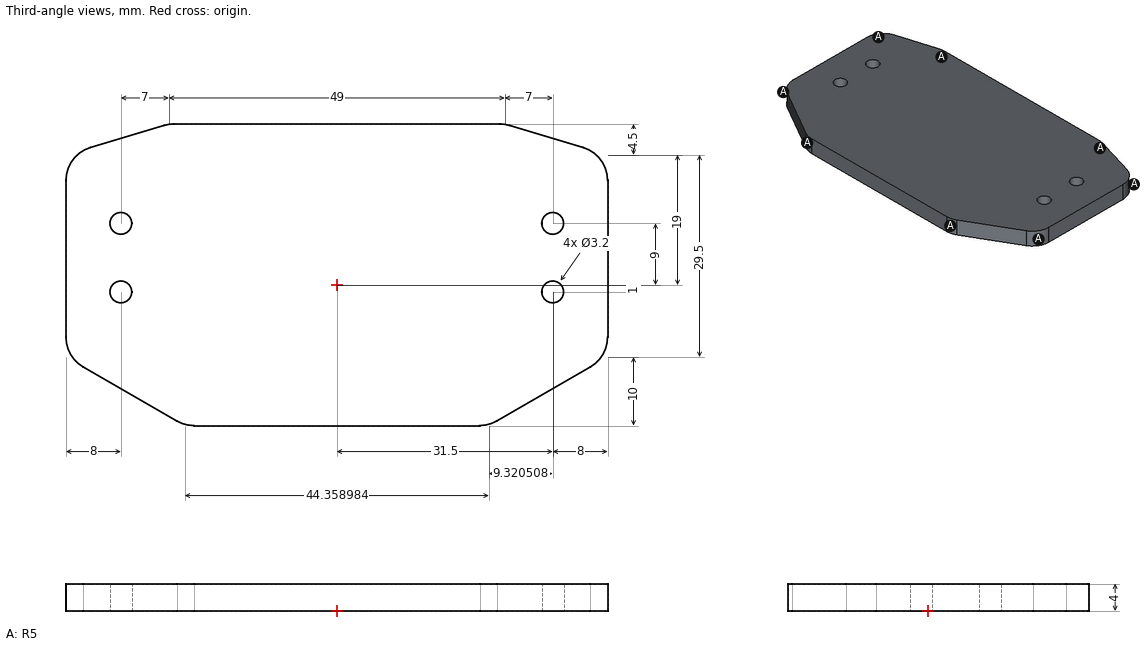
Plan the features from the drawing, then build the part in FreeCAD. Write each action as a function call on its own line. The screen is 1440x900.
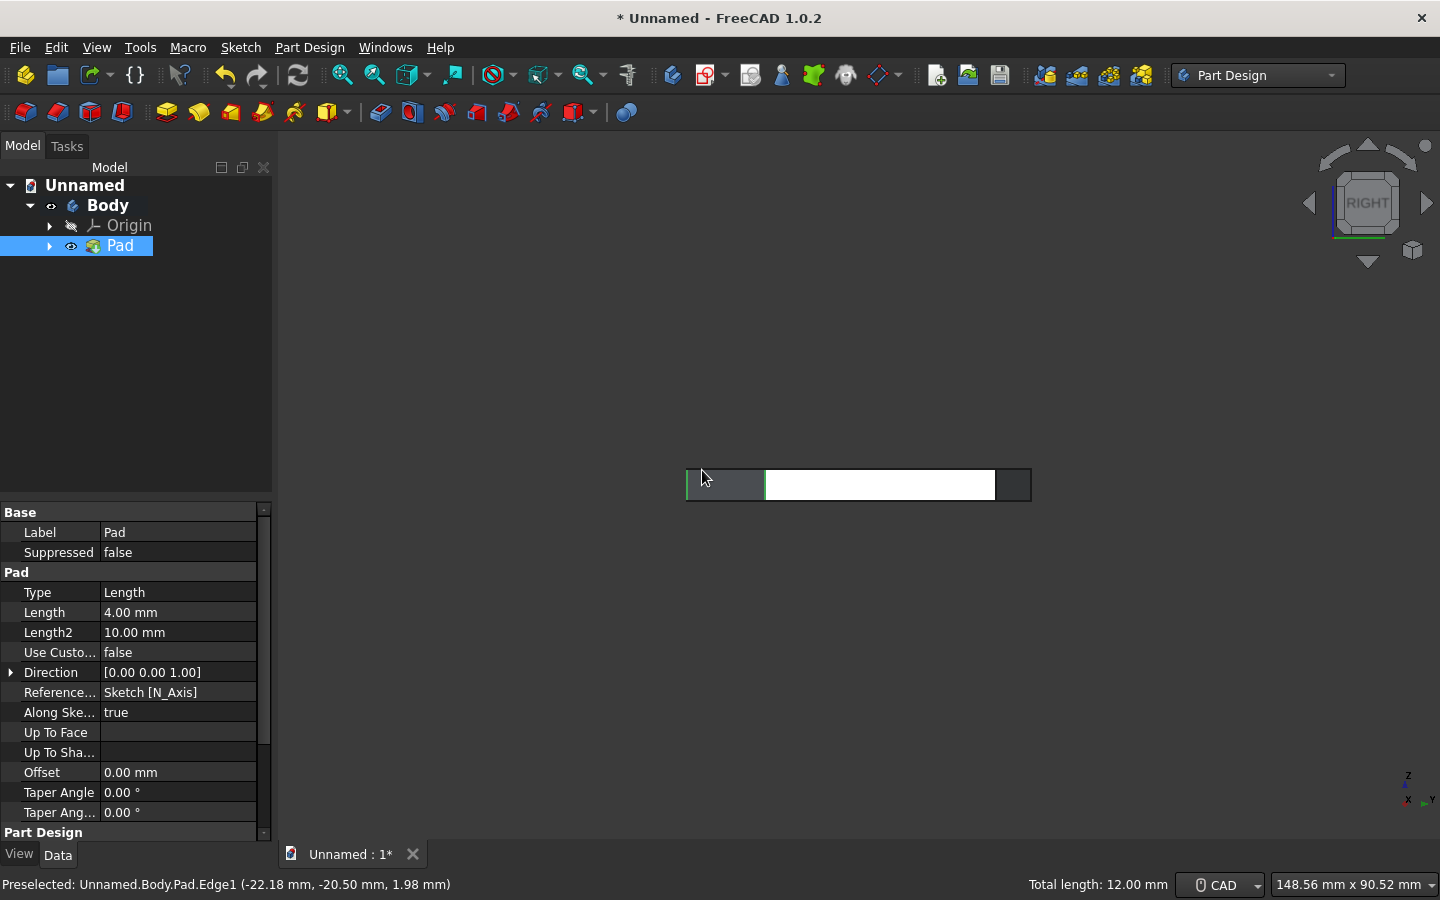
click(996, 484, ctrl)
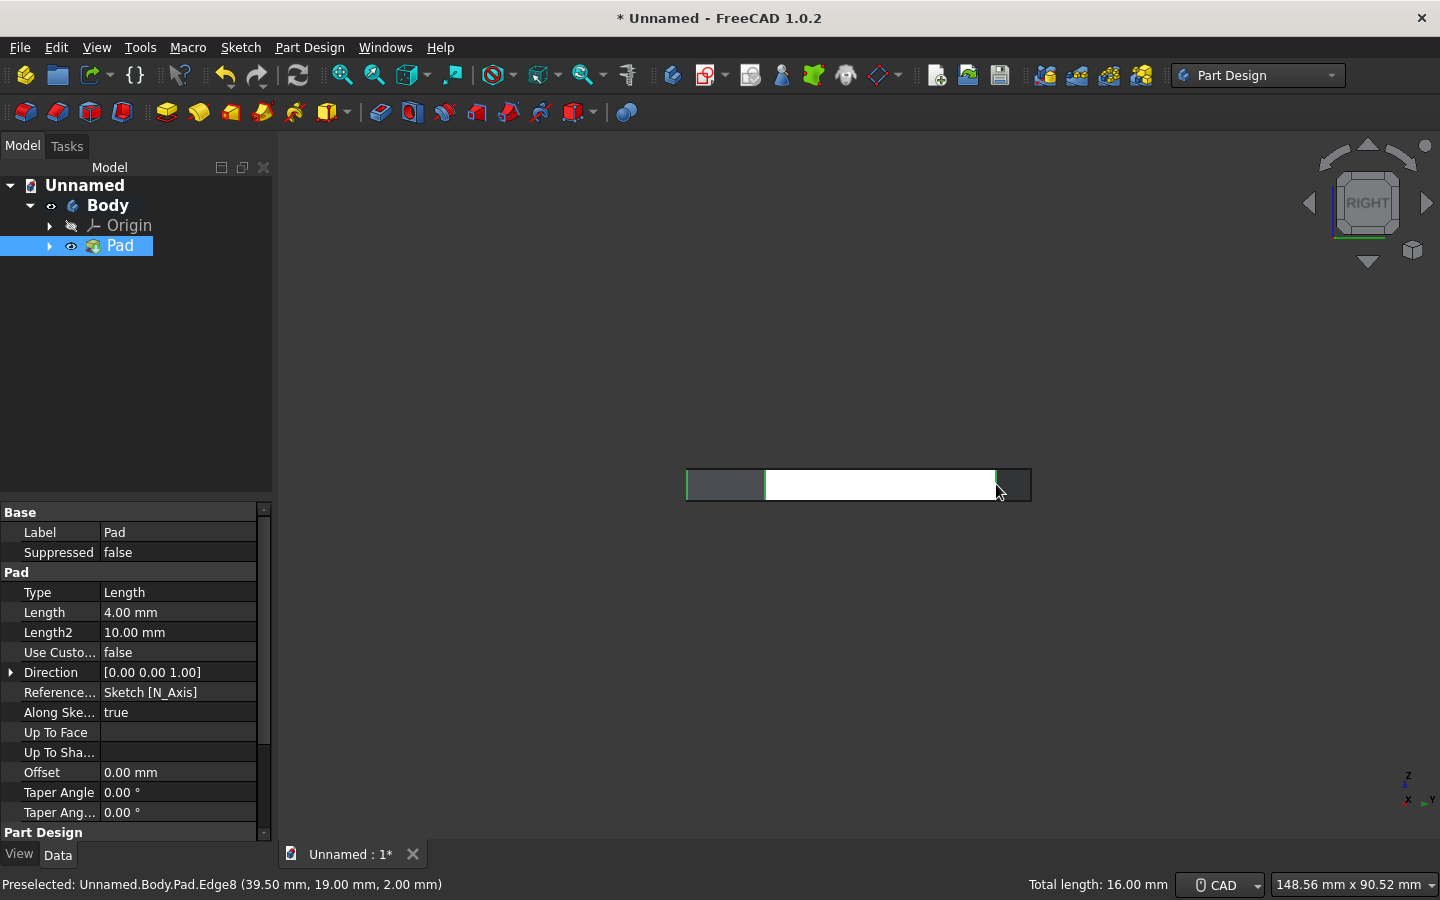
key(5)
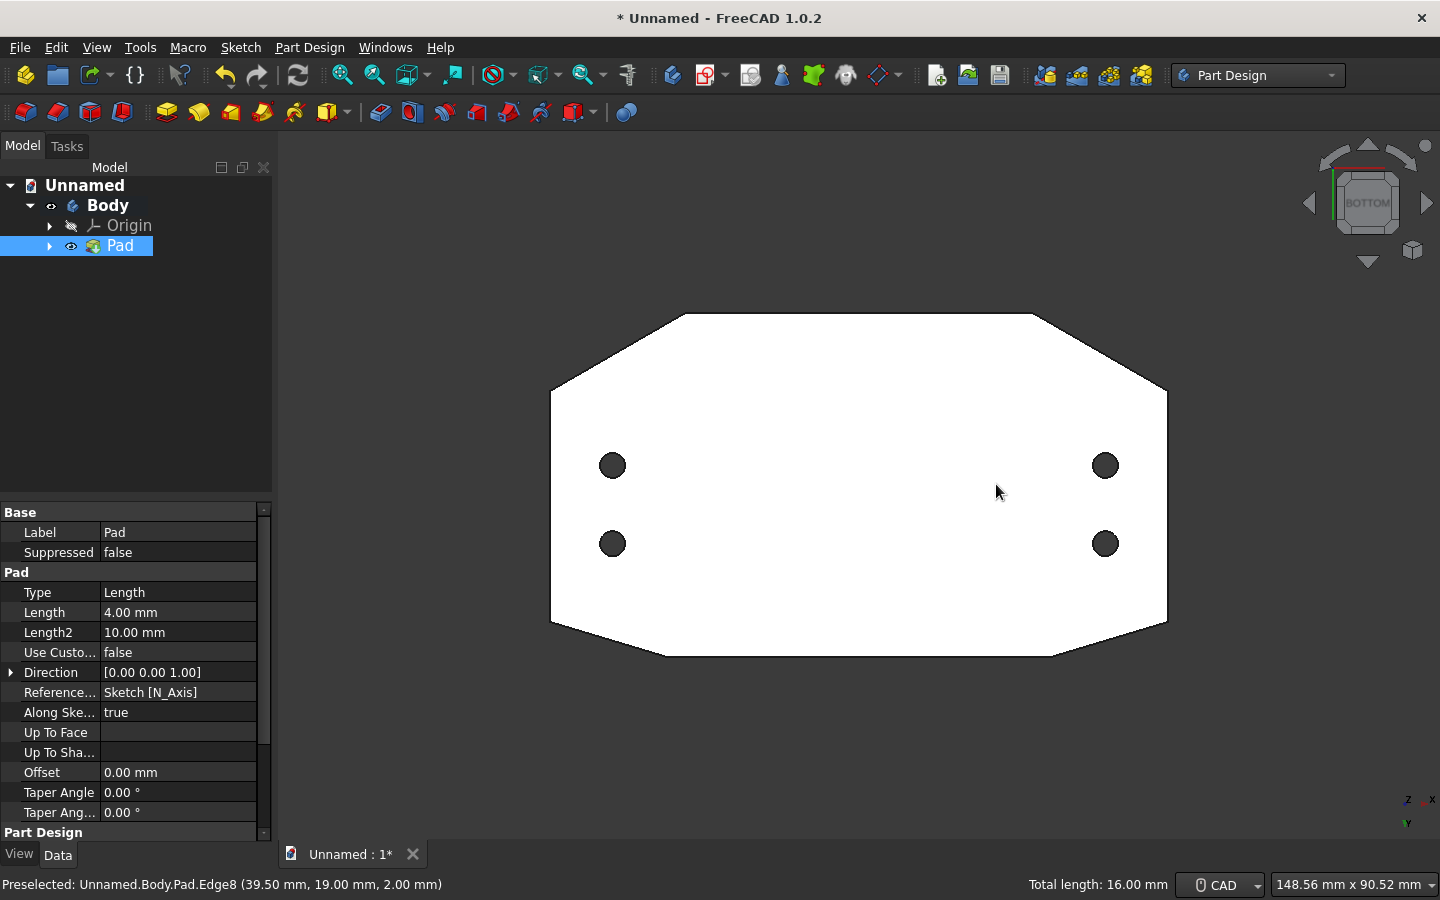
key(4)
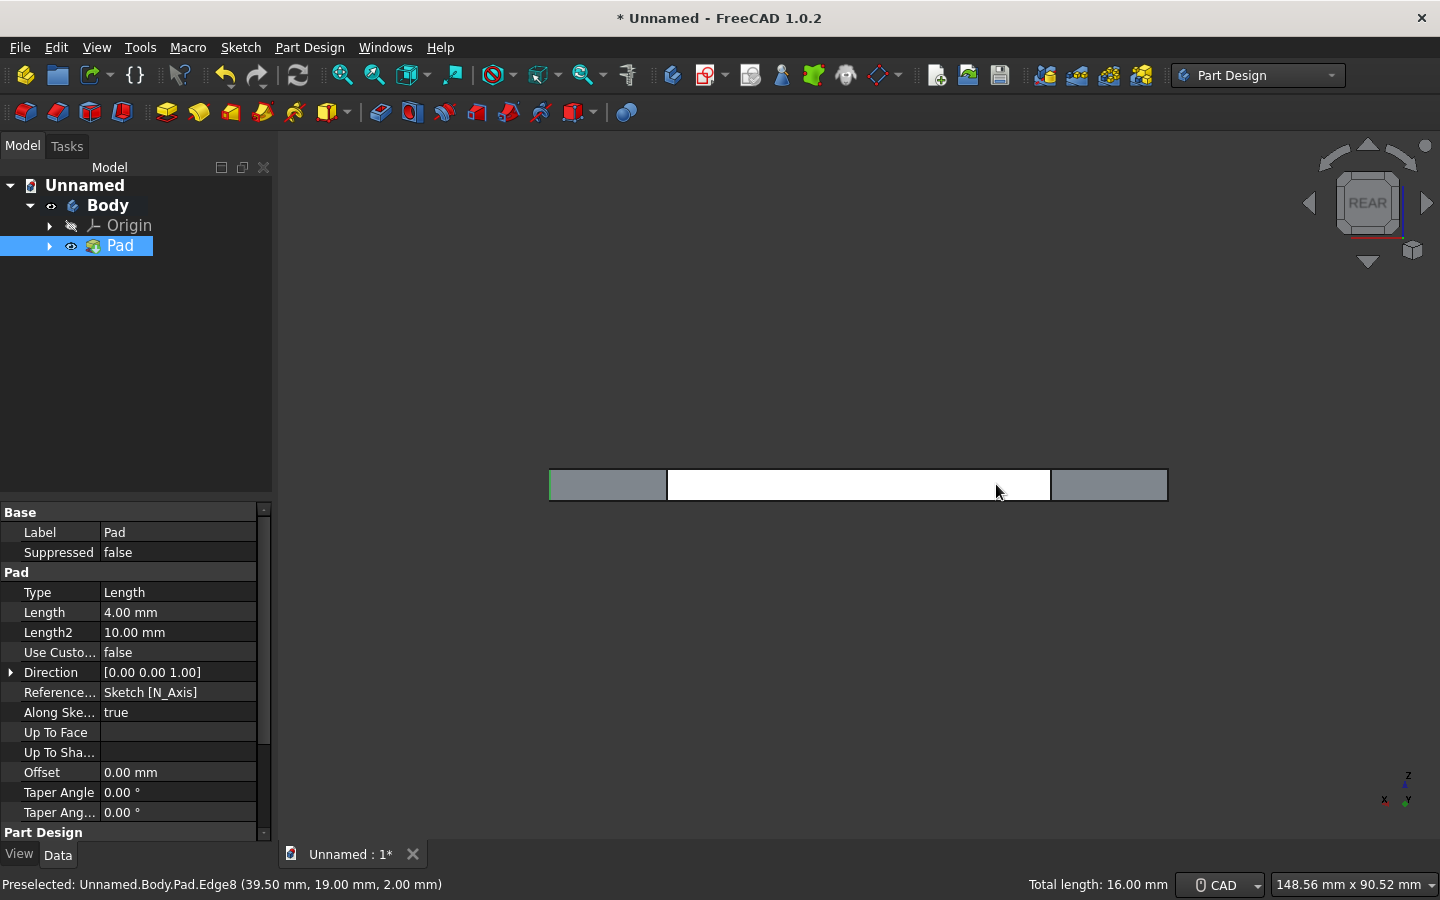
click(1051, 484, ctrl)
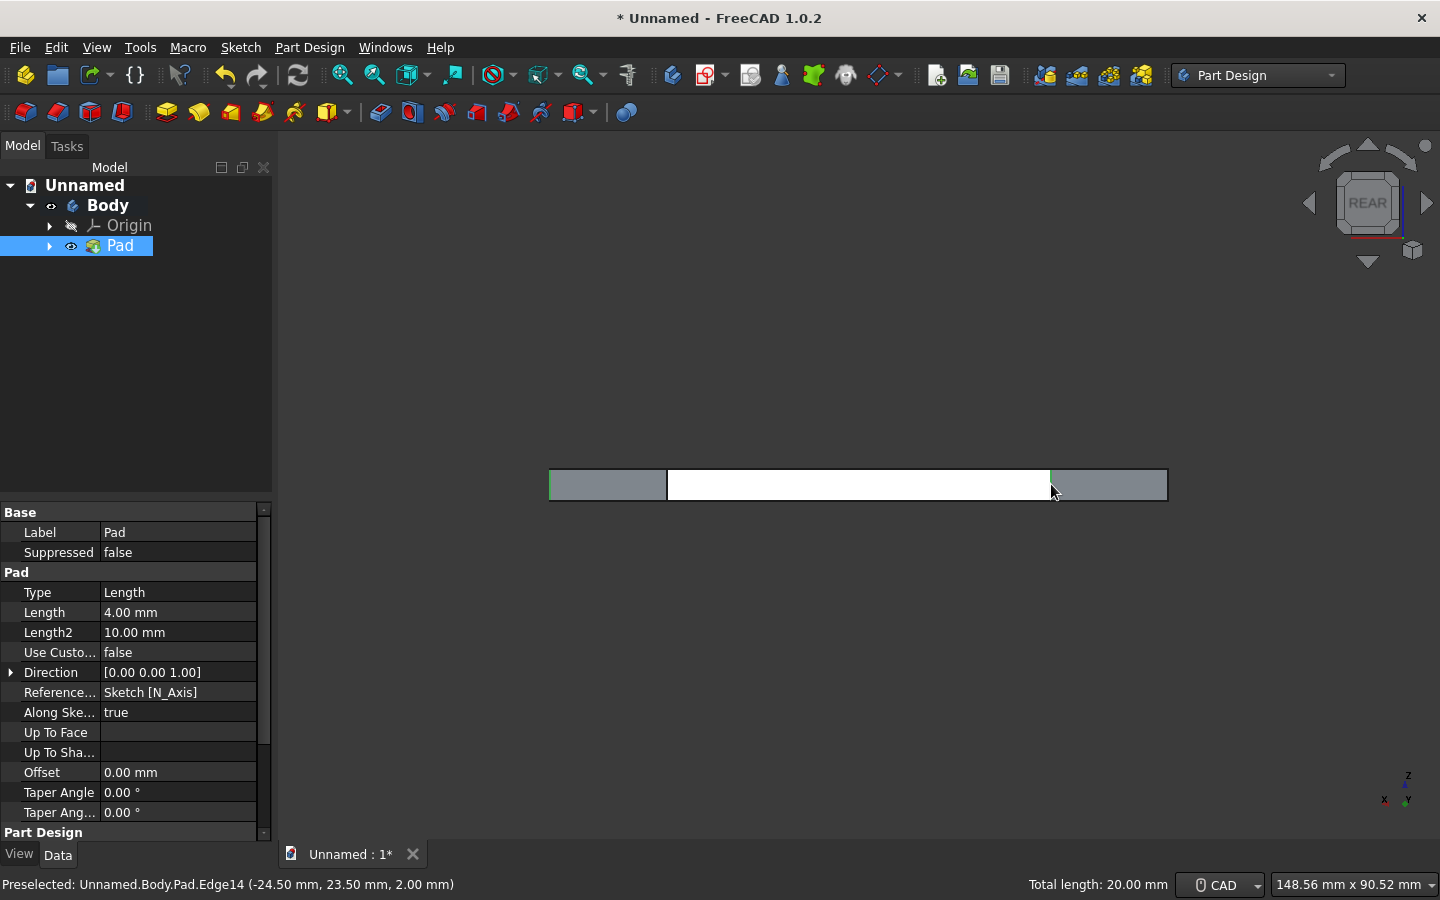
click(667, 484, ctrl)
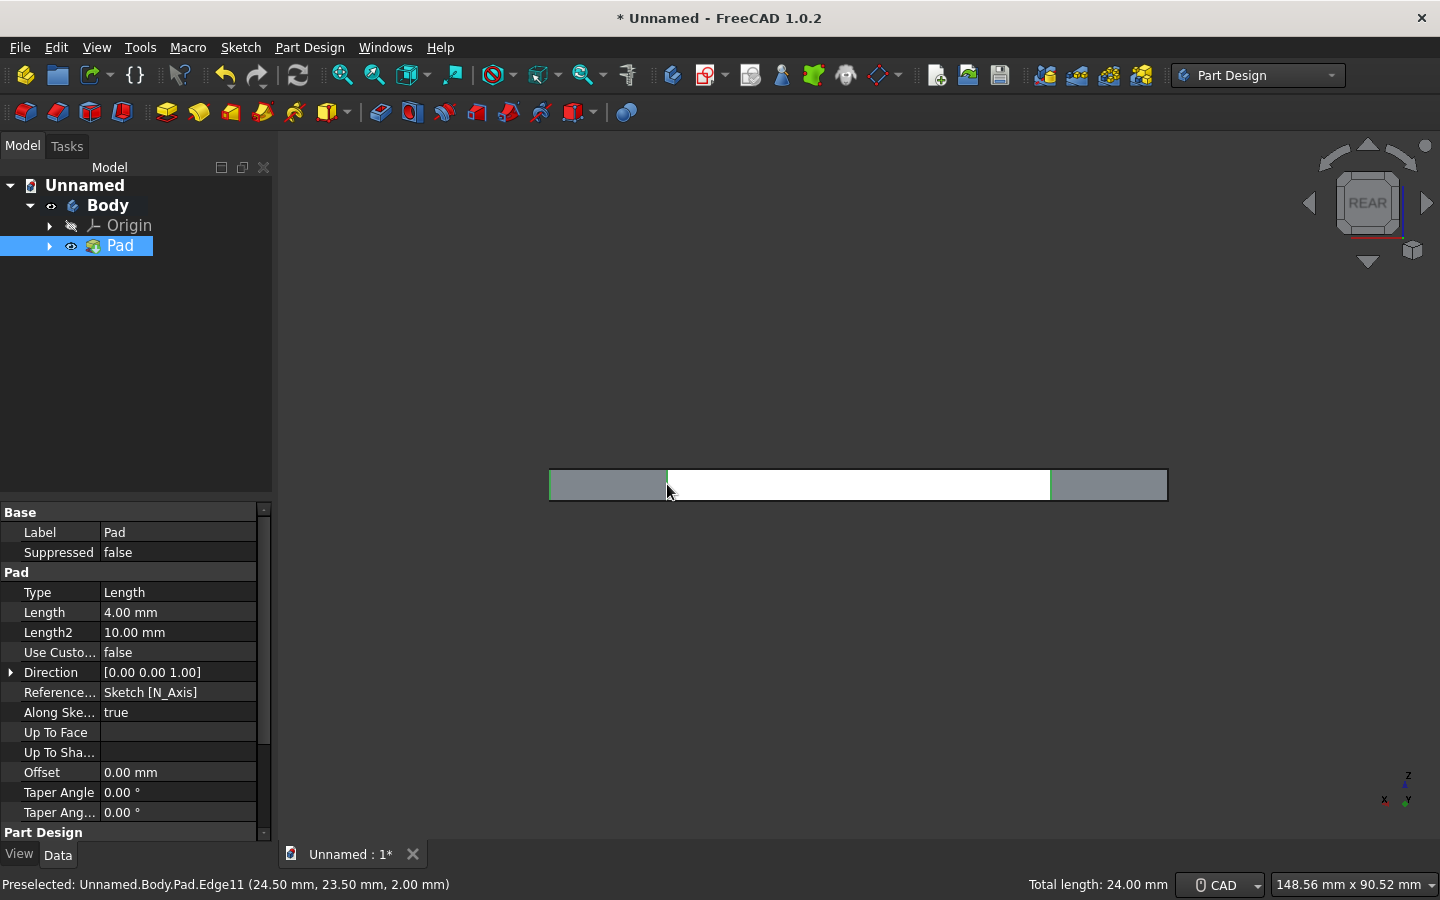
key(6)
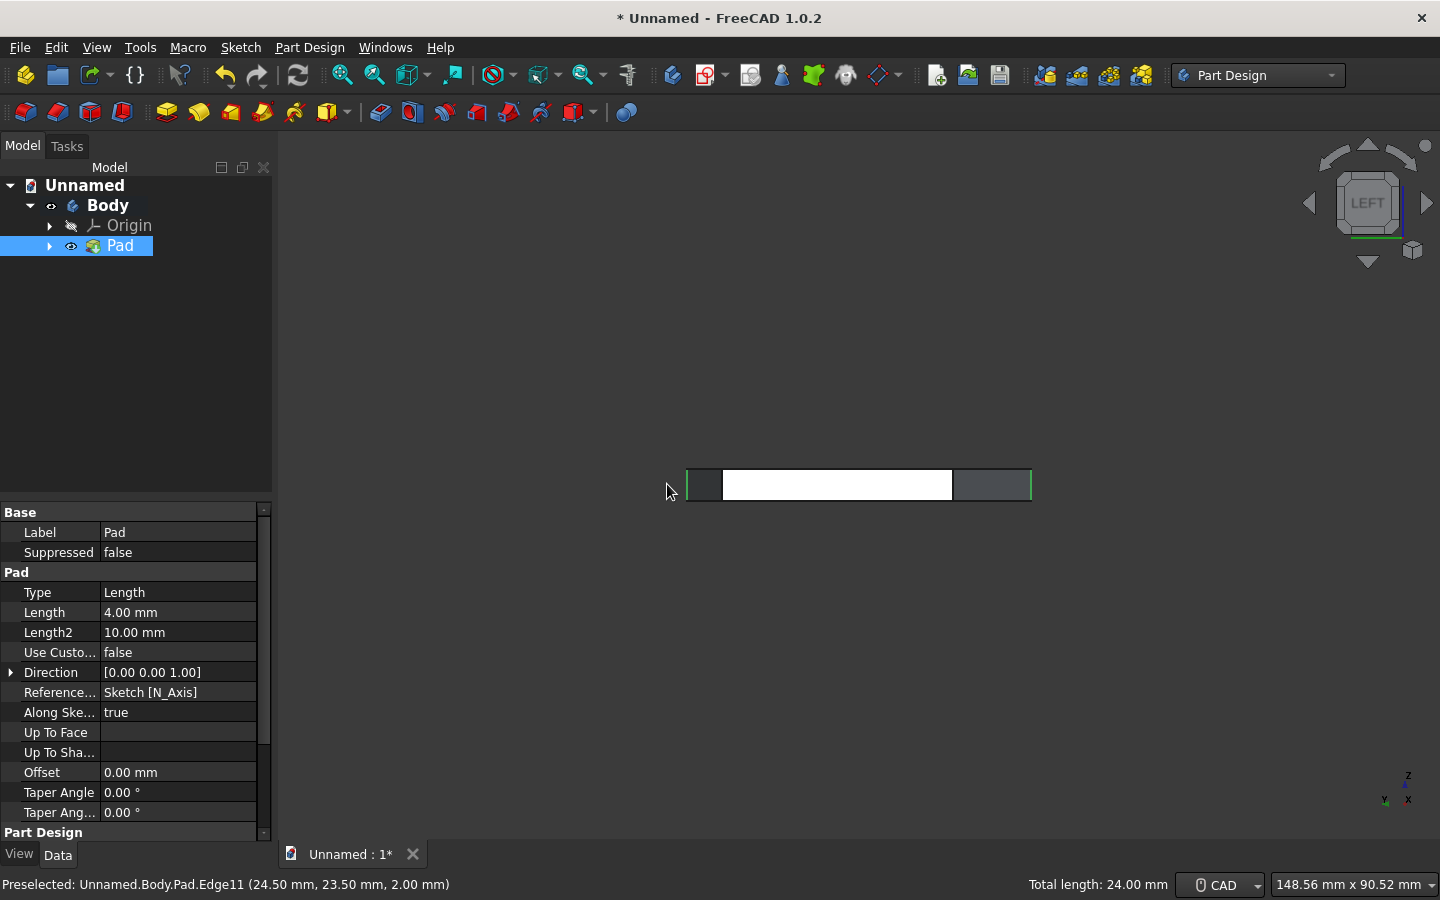
key(v)
key(f)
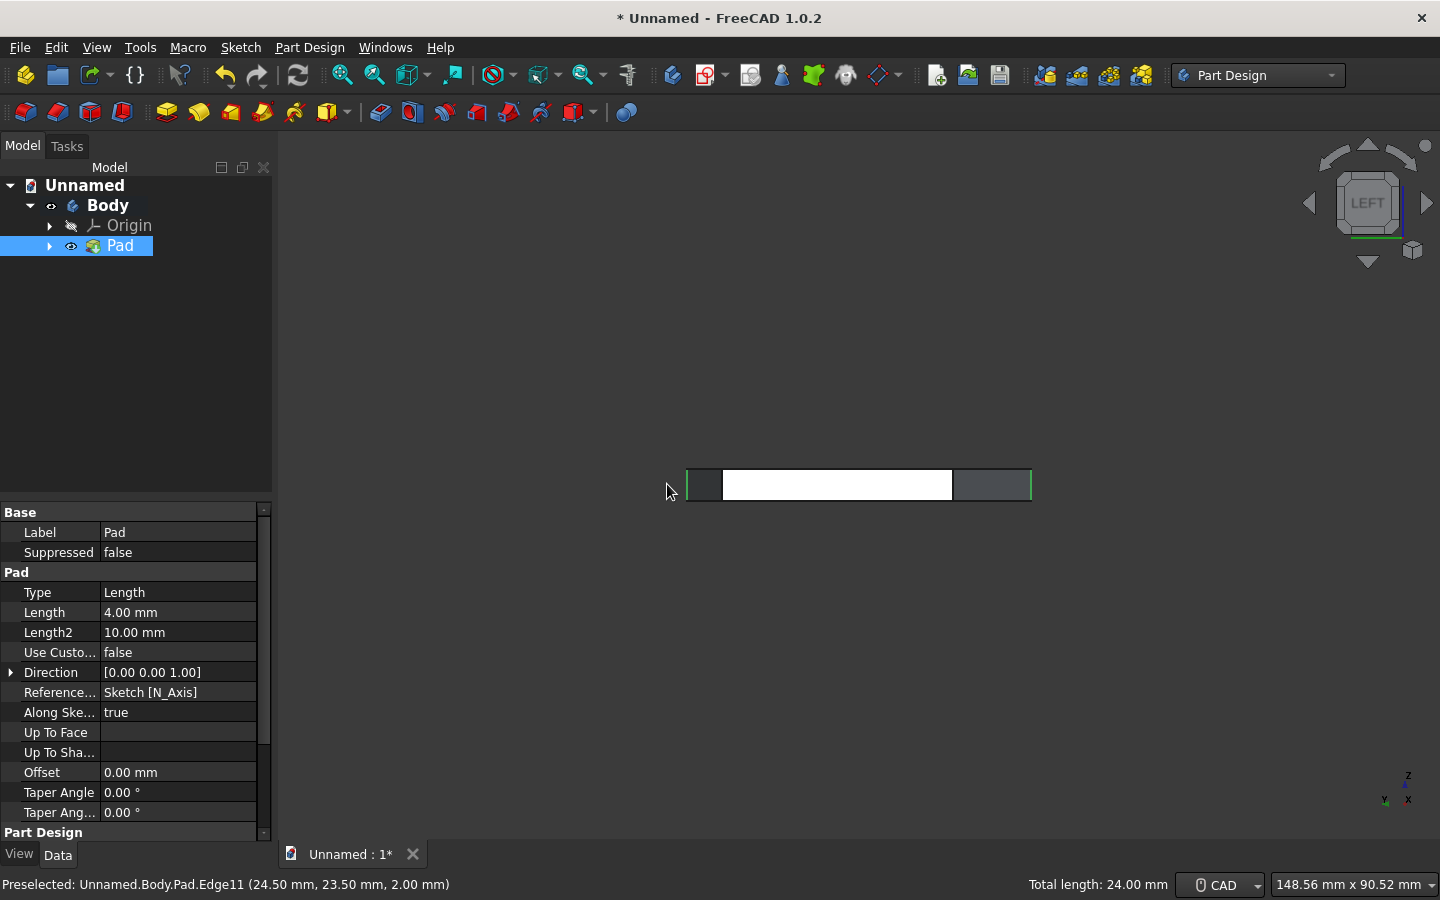
click(953, 484, ctrl)